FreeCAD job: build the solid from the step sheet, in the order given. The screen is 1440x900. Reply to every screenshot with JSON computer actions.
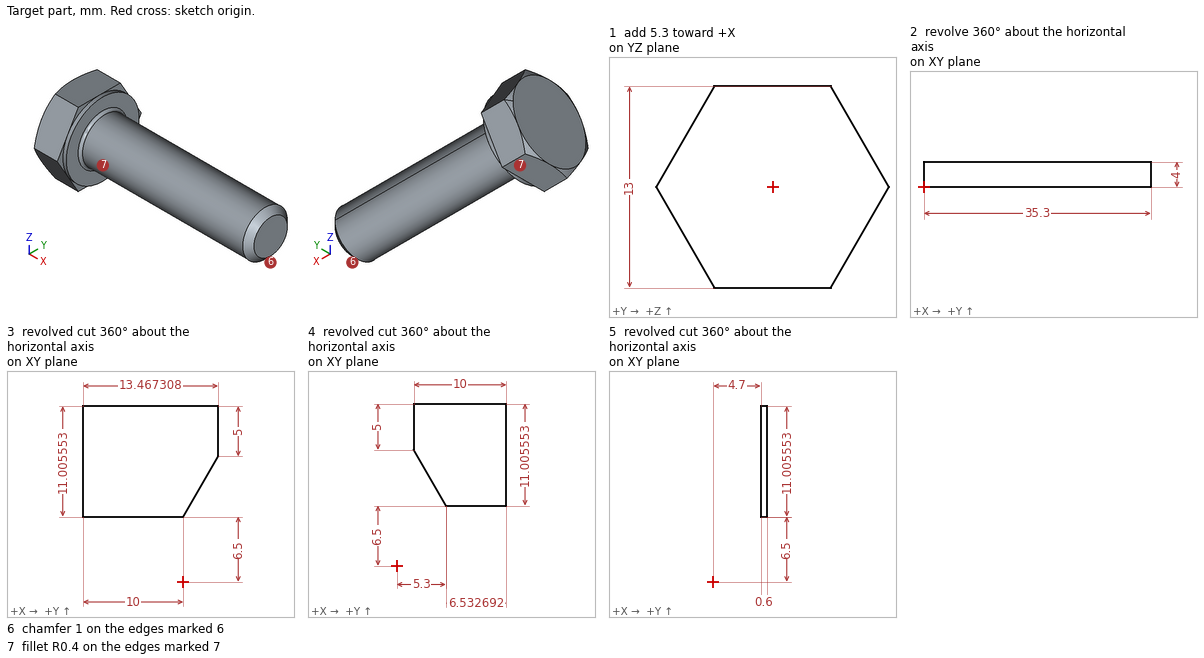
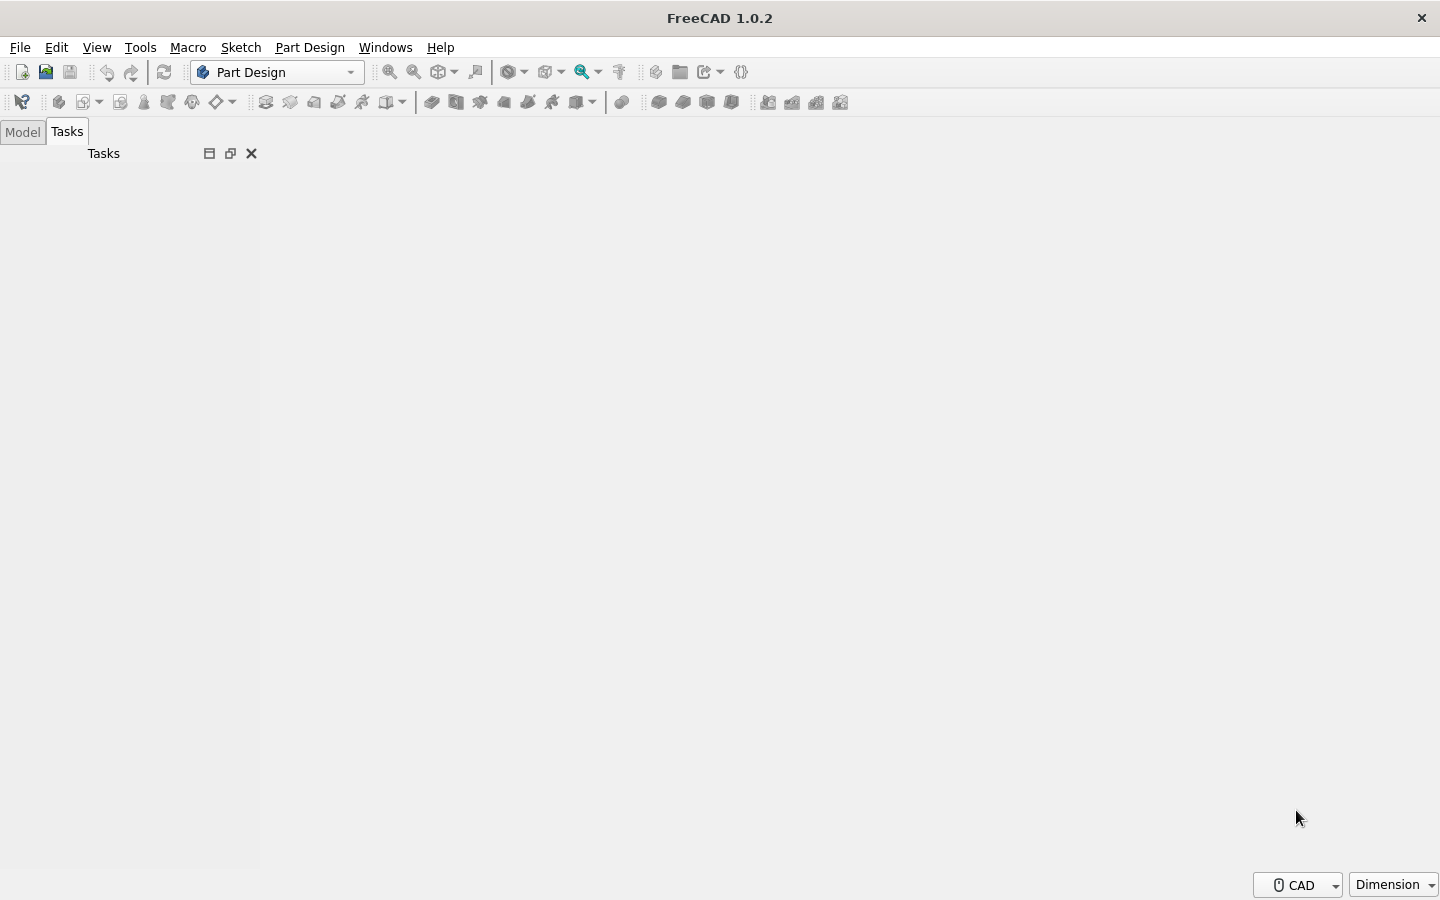
{"action": "key", "text": "ctrl+n"}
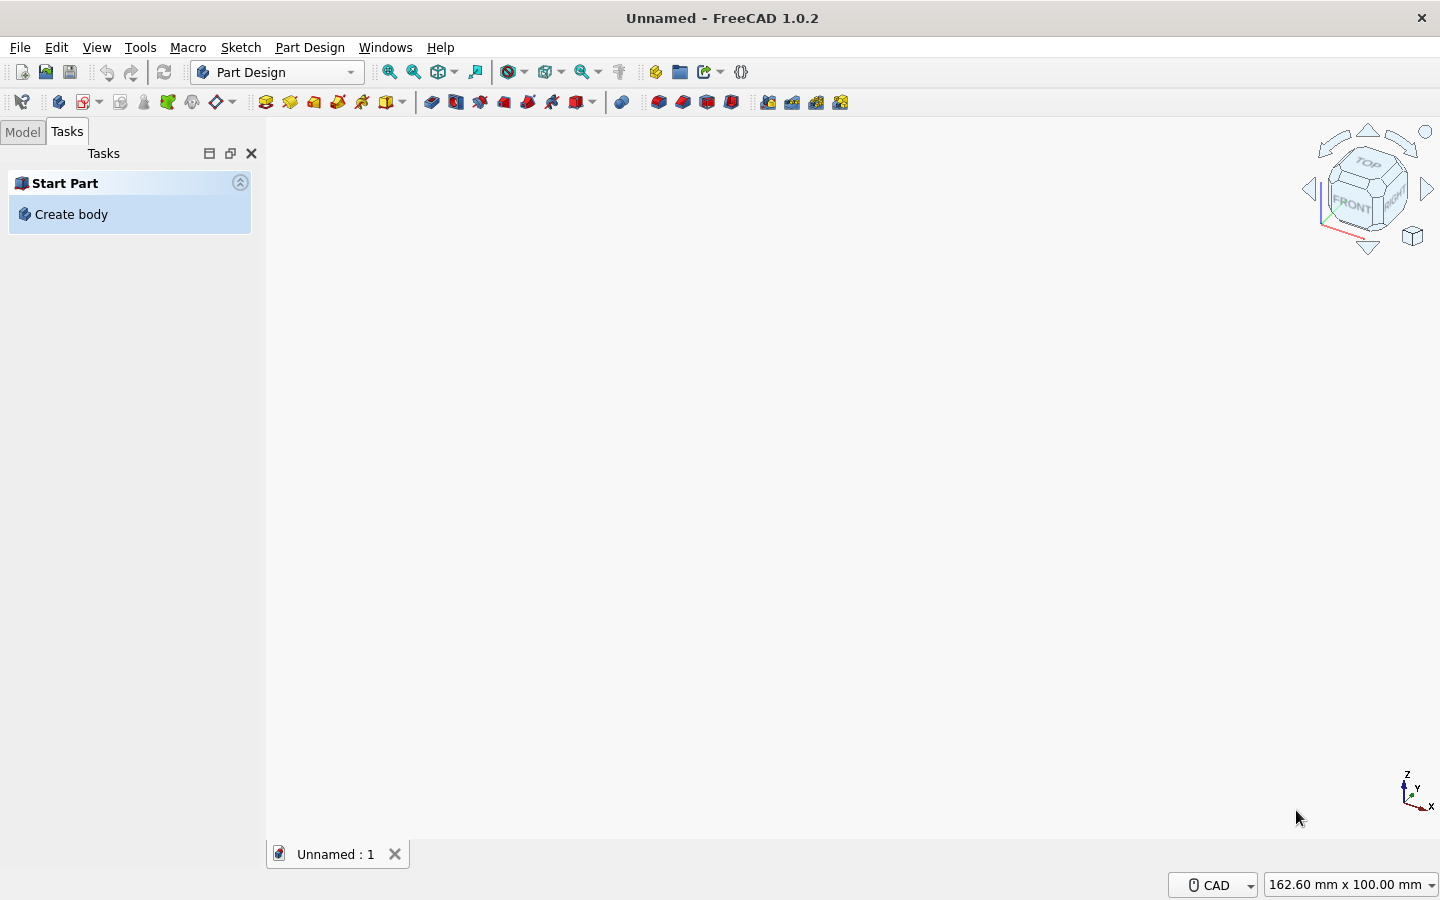
{"action": "left_click", "coordinate": [84, 102]}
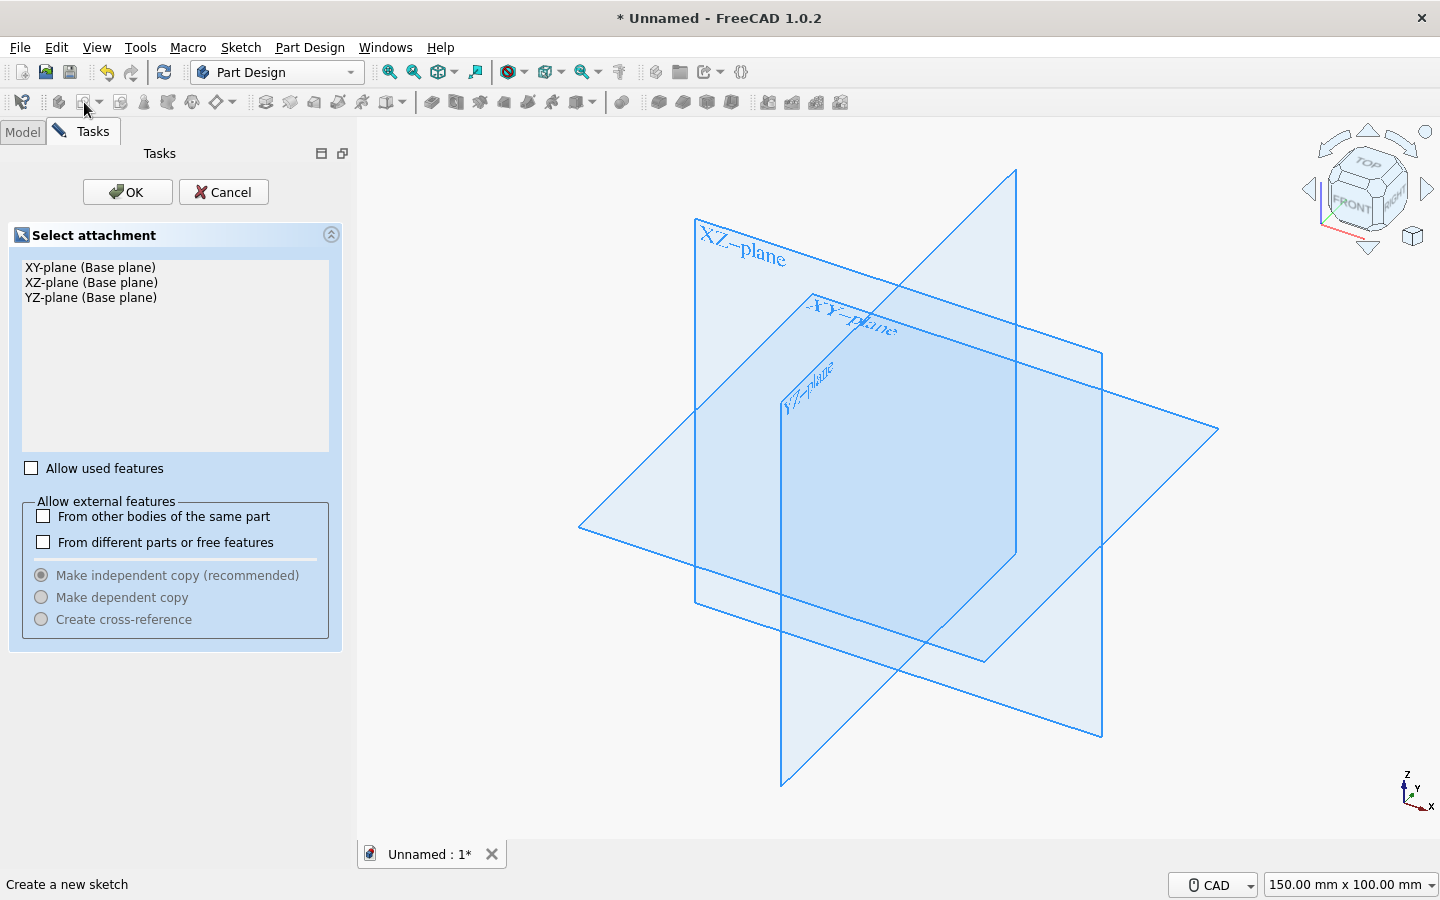
{"action": "left_click", "coordinate": [82, 298]}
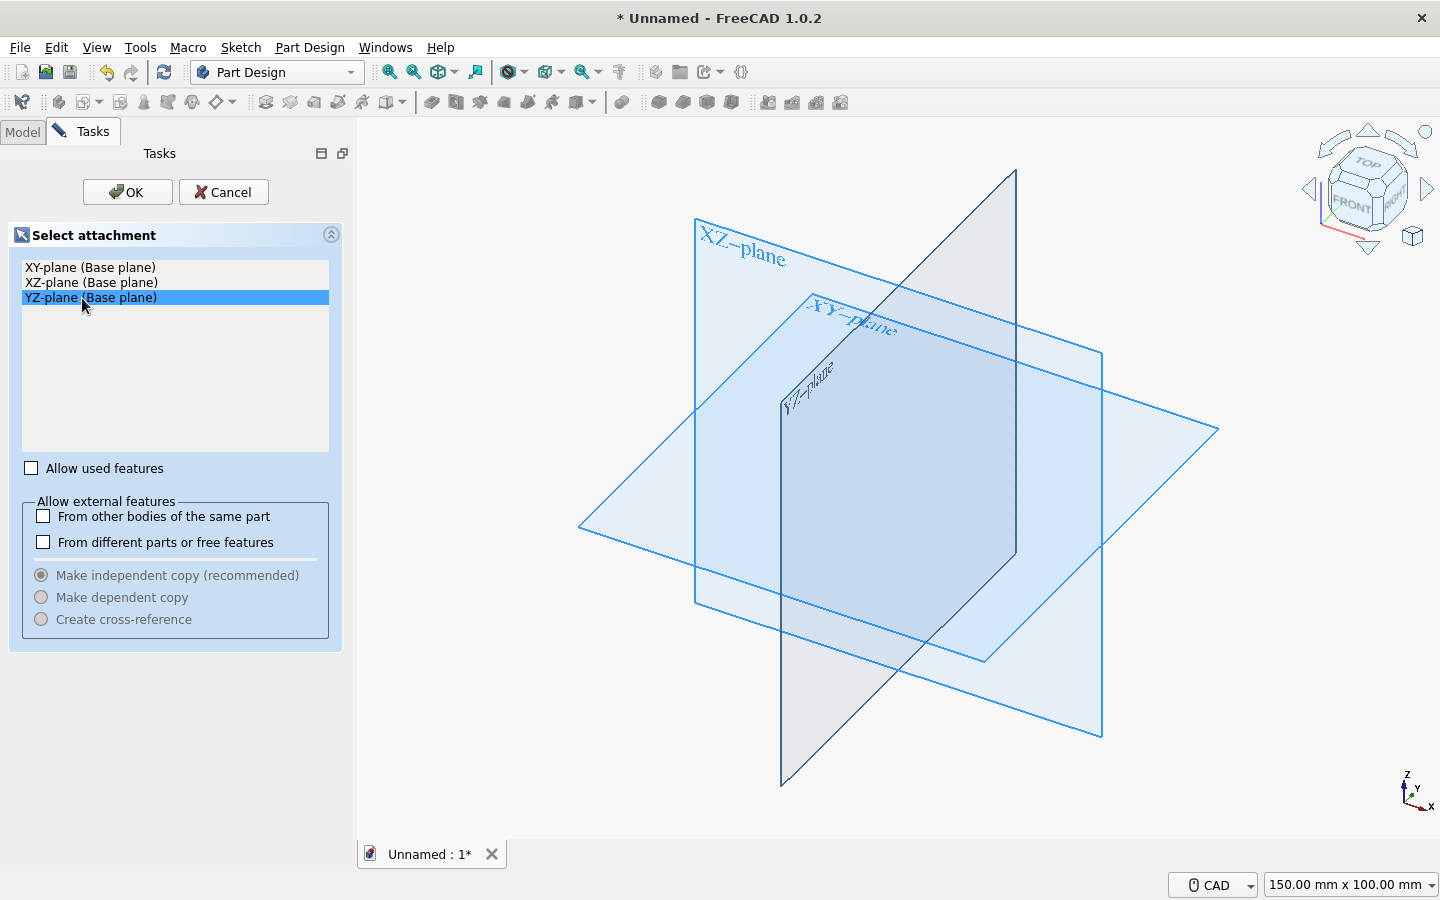
{"action": "left_click", "coordinate": [128, 192]}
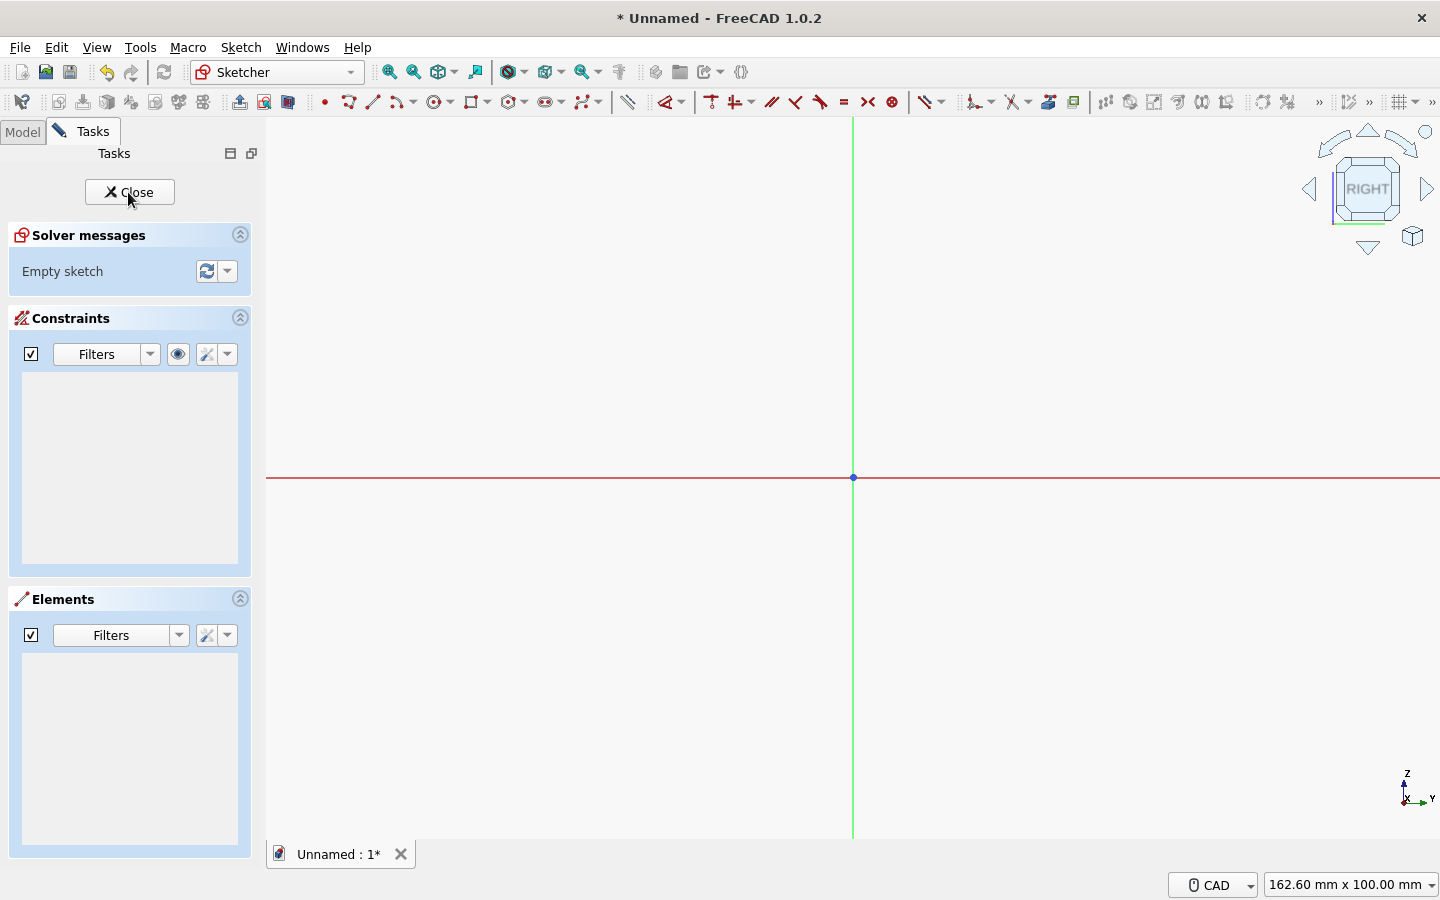
{"action": "scroll", "coordinate": [870, 478], "scroll_direction": "up", "scroll_amount": 8}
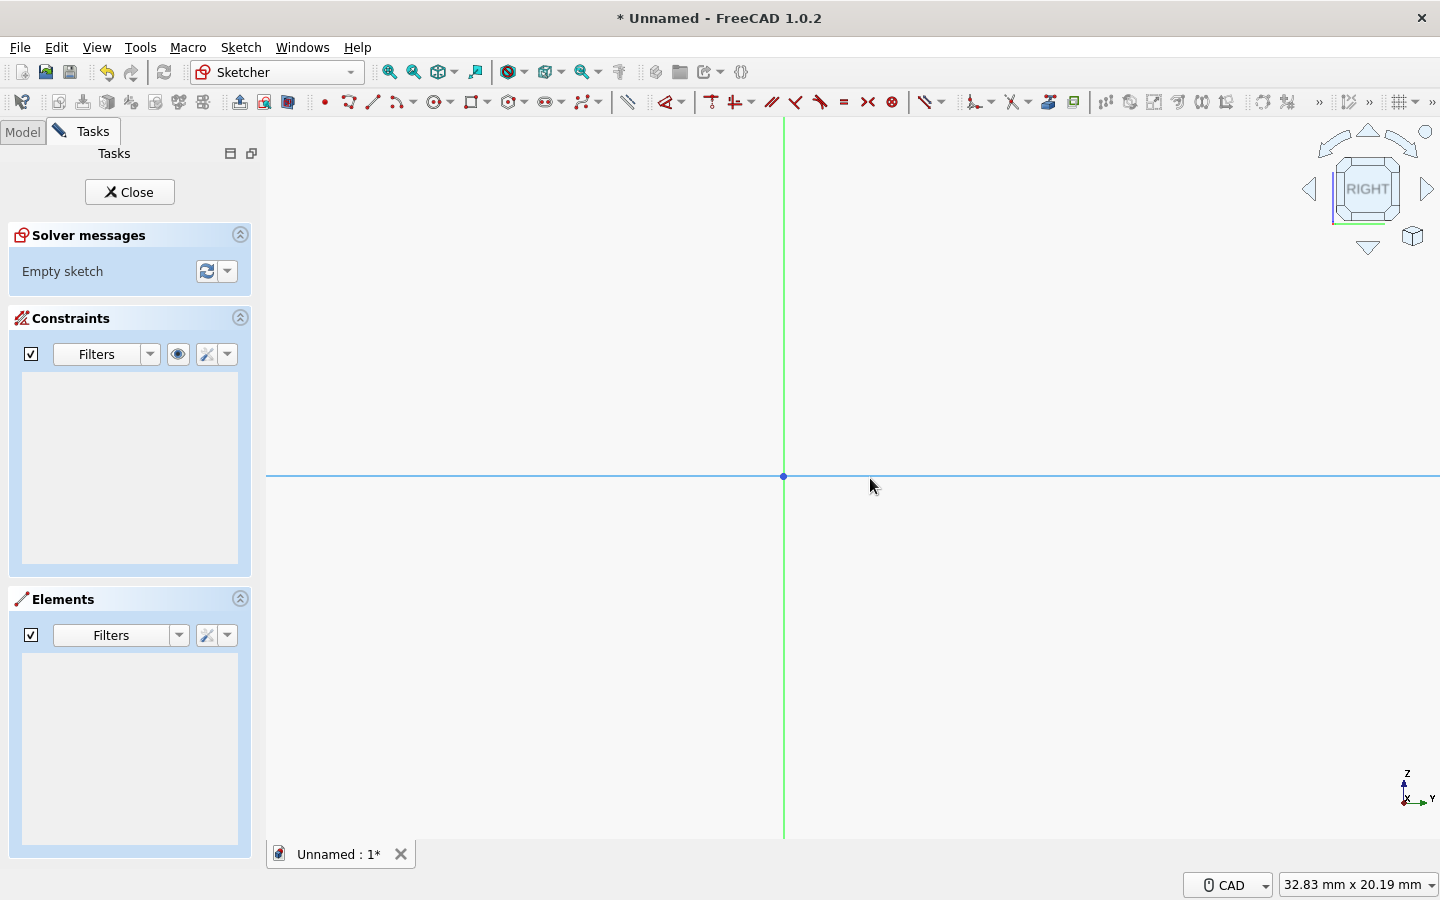
{"action": "key", "text": "g p 6"}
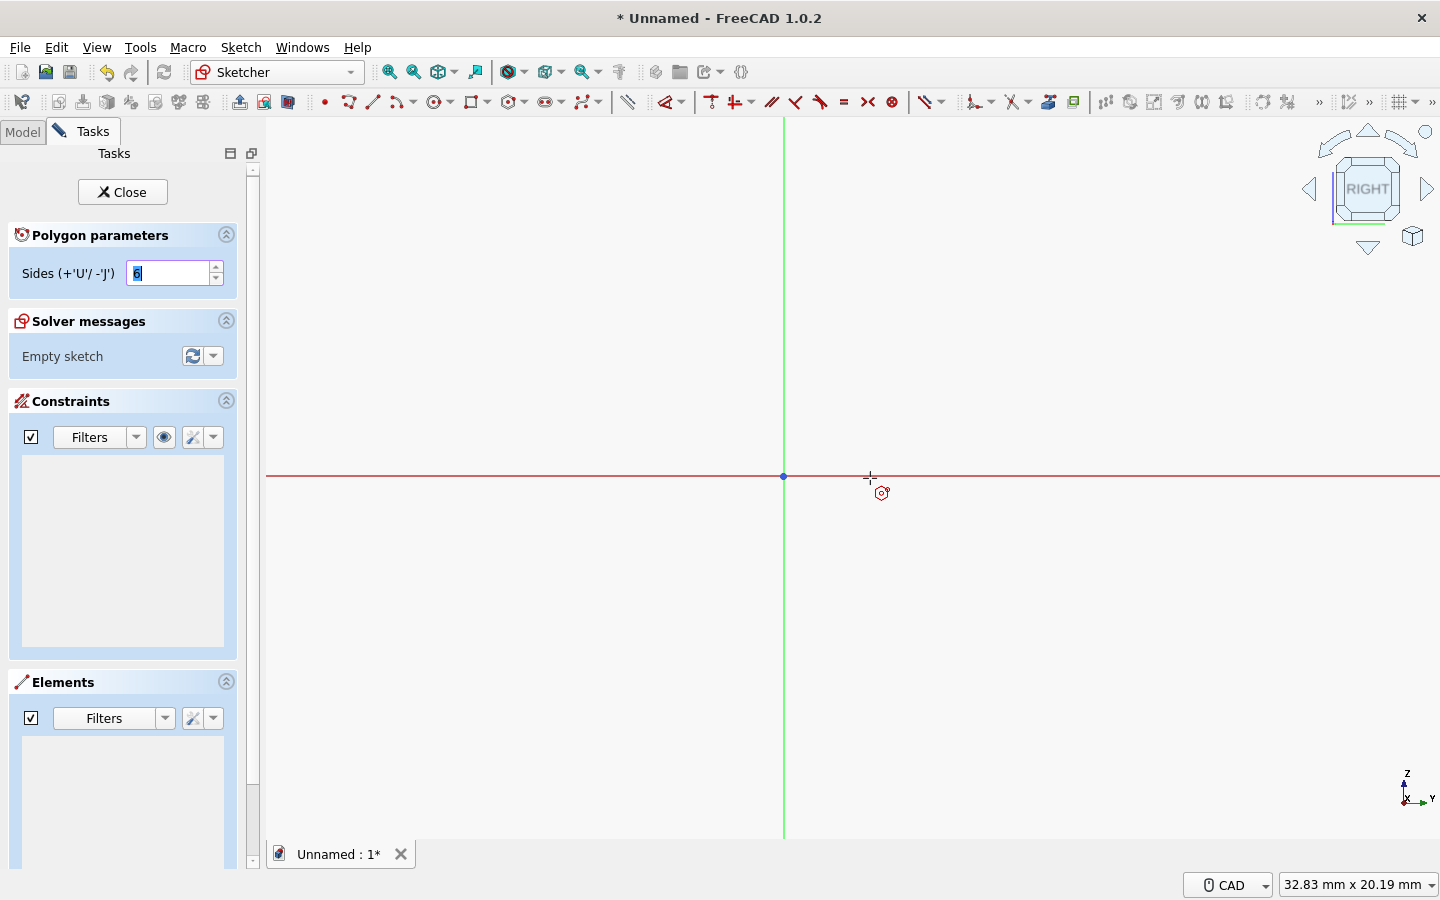
{"action": "left_click", "coordinate": [784, 476]}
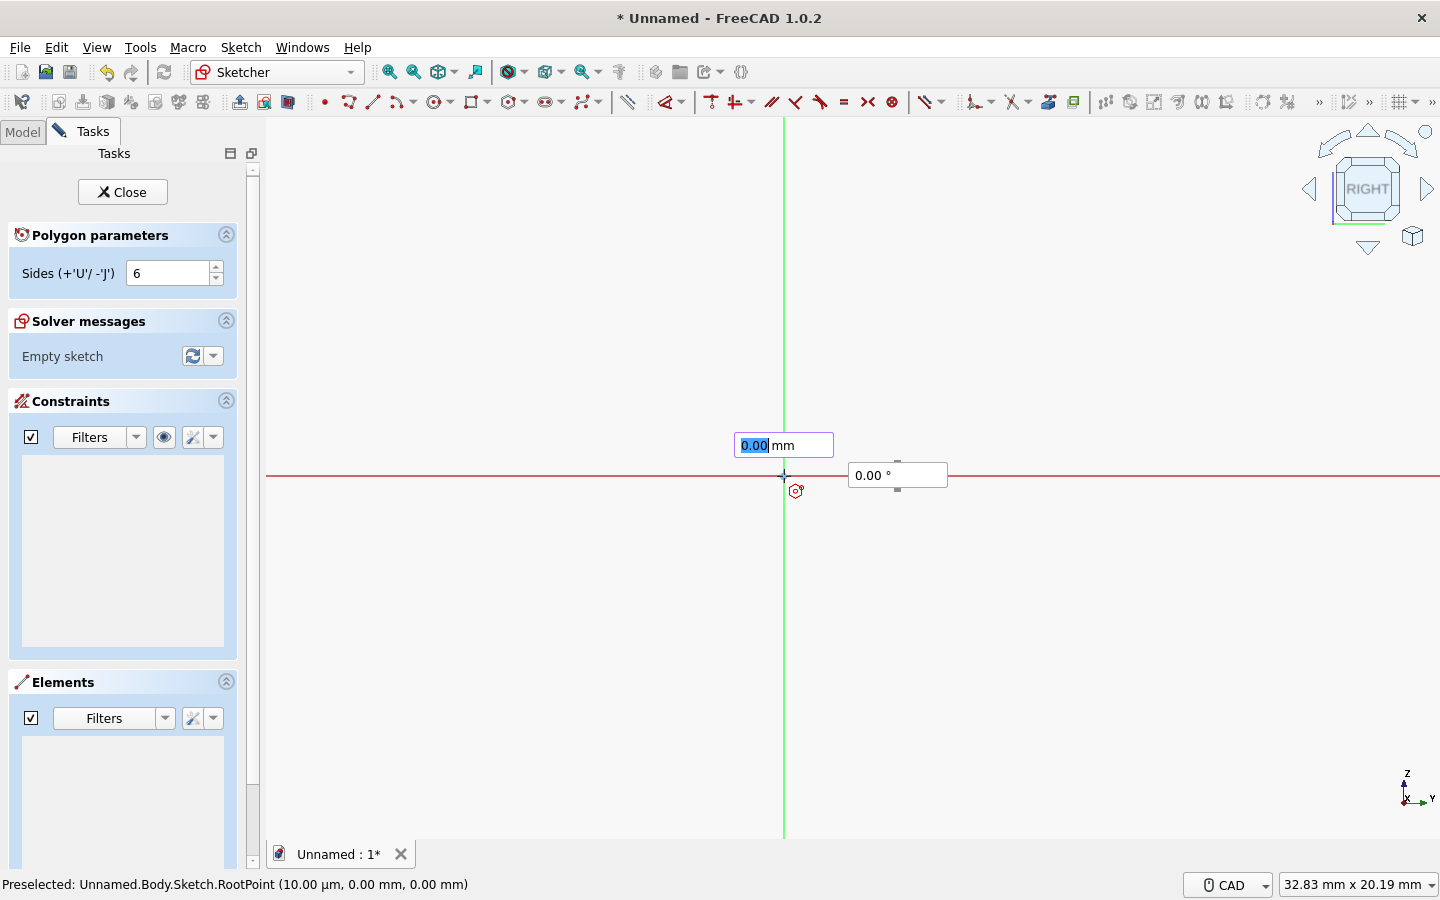
{"action": "left_click", "coordinate": [1052, 476]}
{"action": "right_click", "coordinate": [1052, 476]}